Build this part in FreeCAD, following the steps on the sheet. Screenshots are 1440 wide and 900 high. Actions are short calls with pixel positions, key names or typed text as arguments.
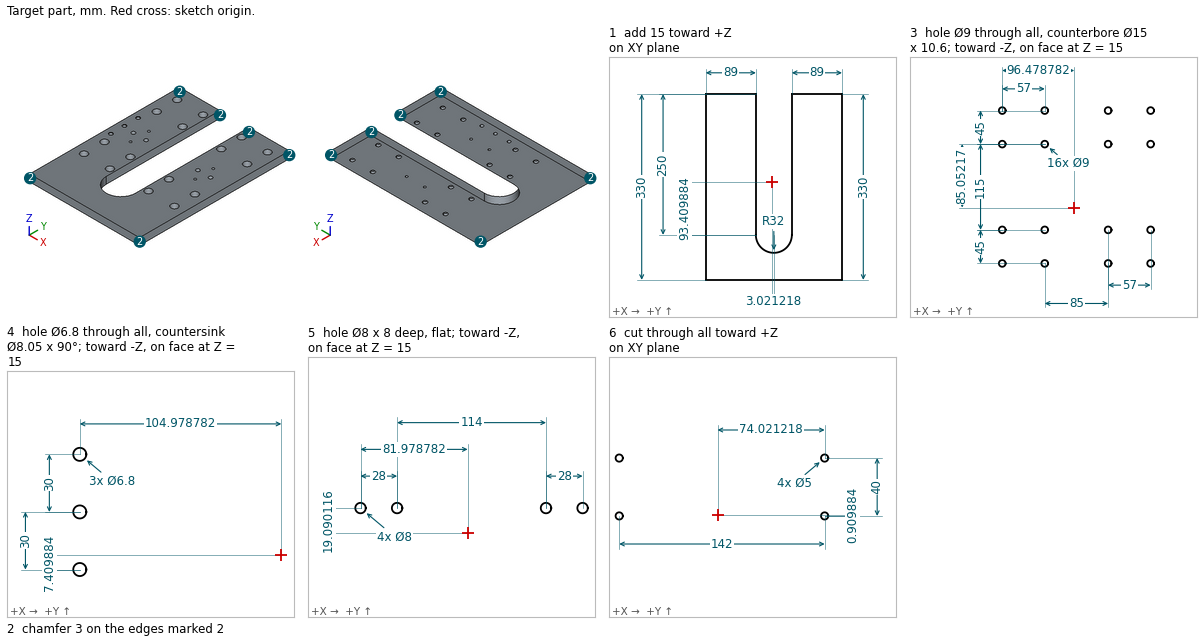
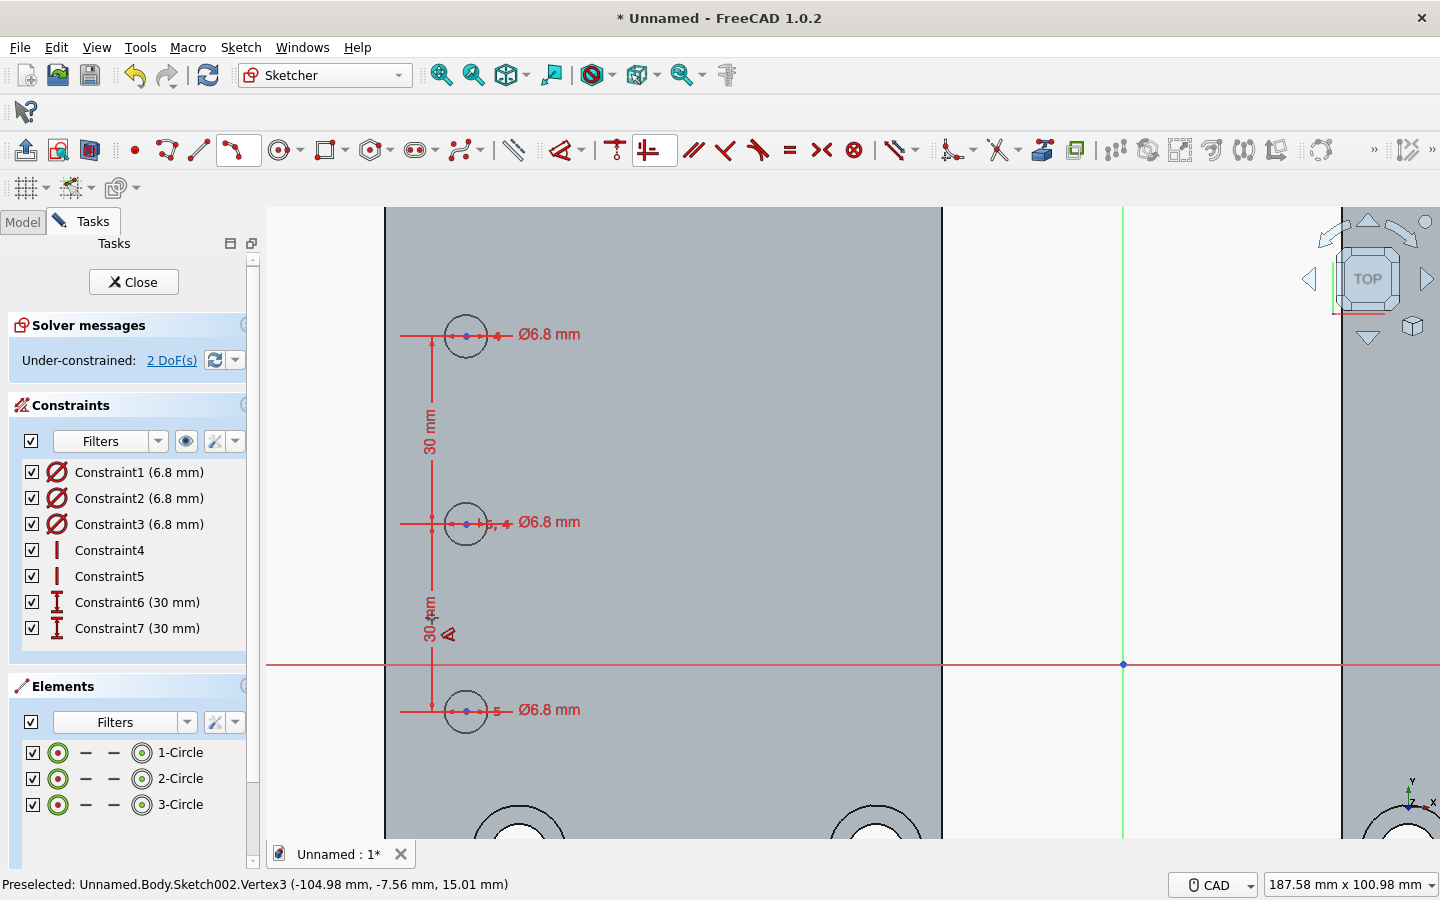
click(466, 712)
click(1157, 688)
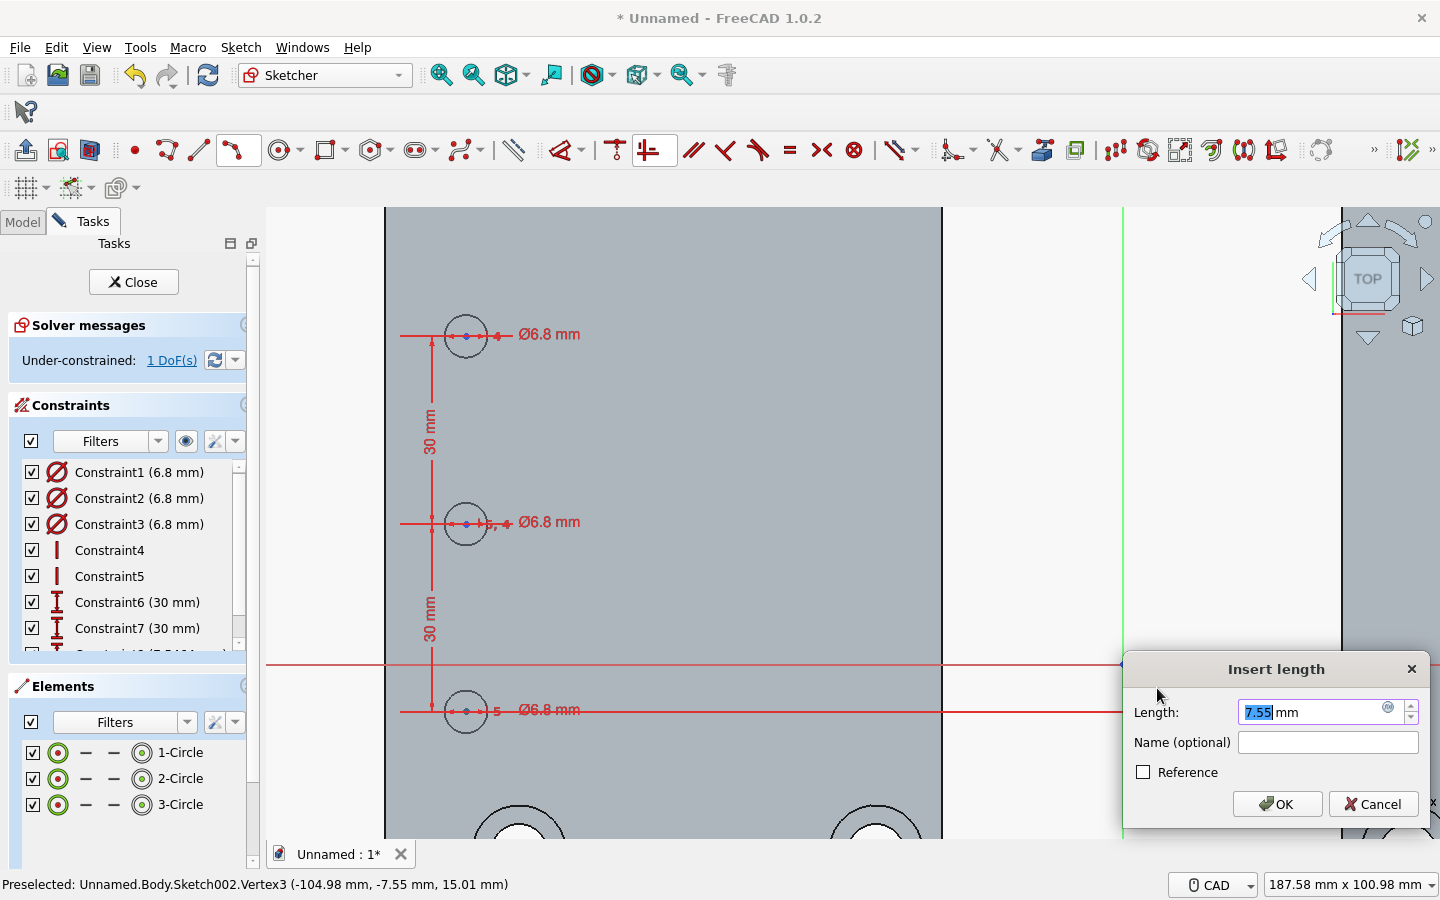
text(7.409884)
key(Return)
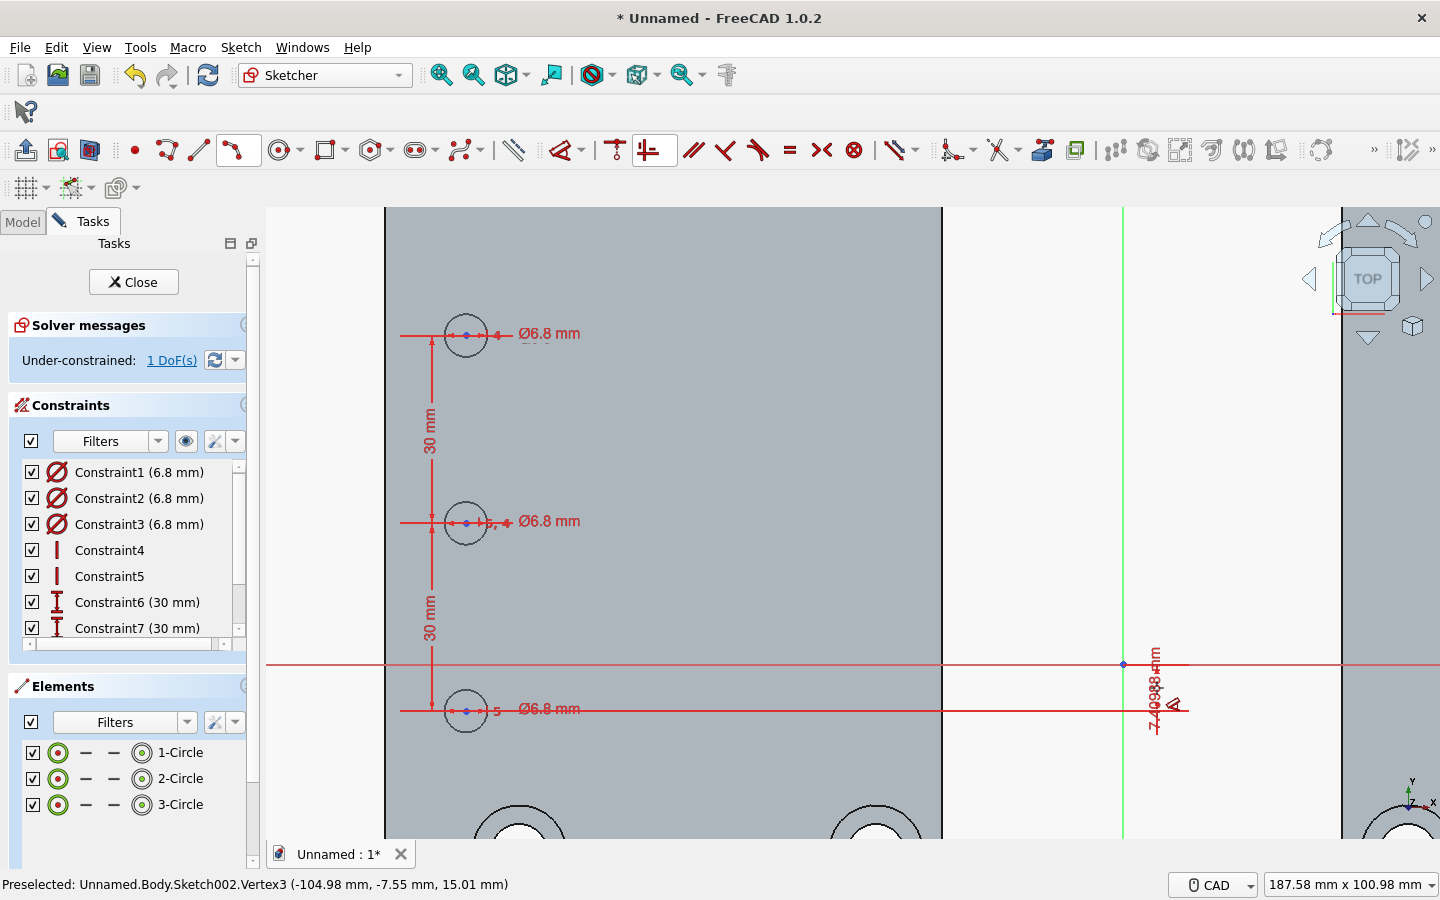
click(466, 336)
click(795, 302)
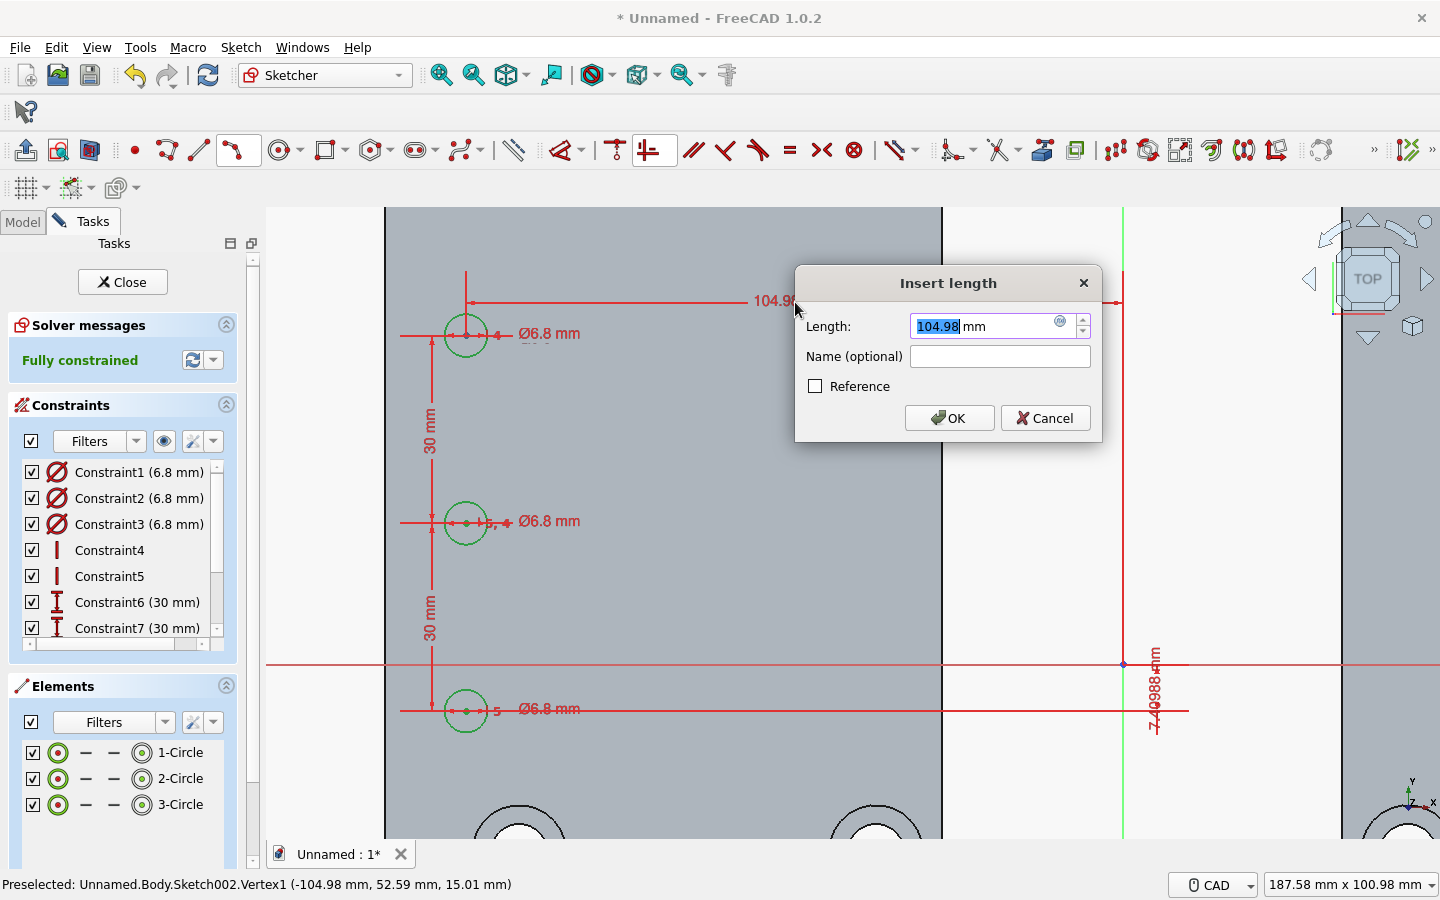
text(104.978782)
key(Return)
key(Escape)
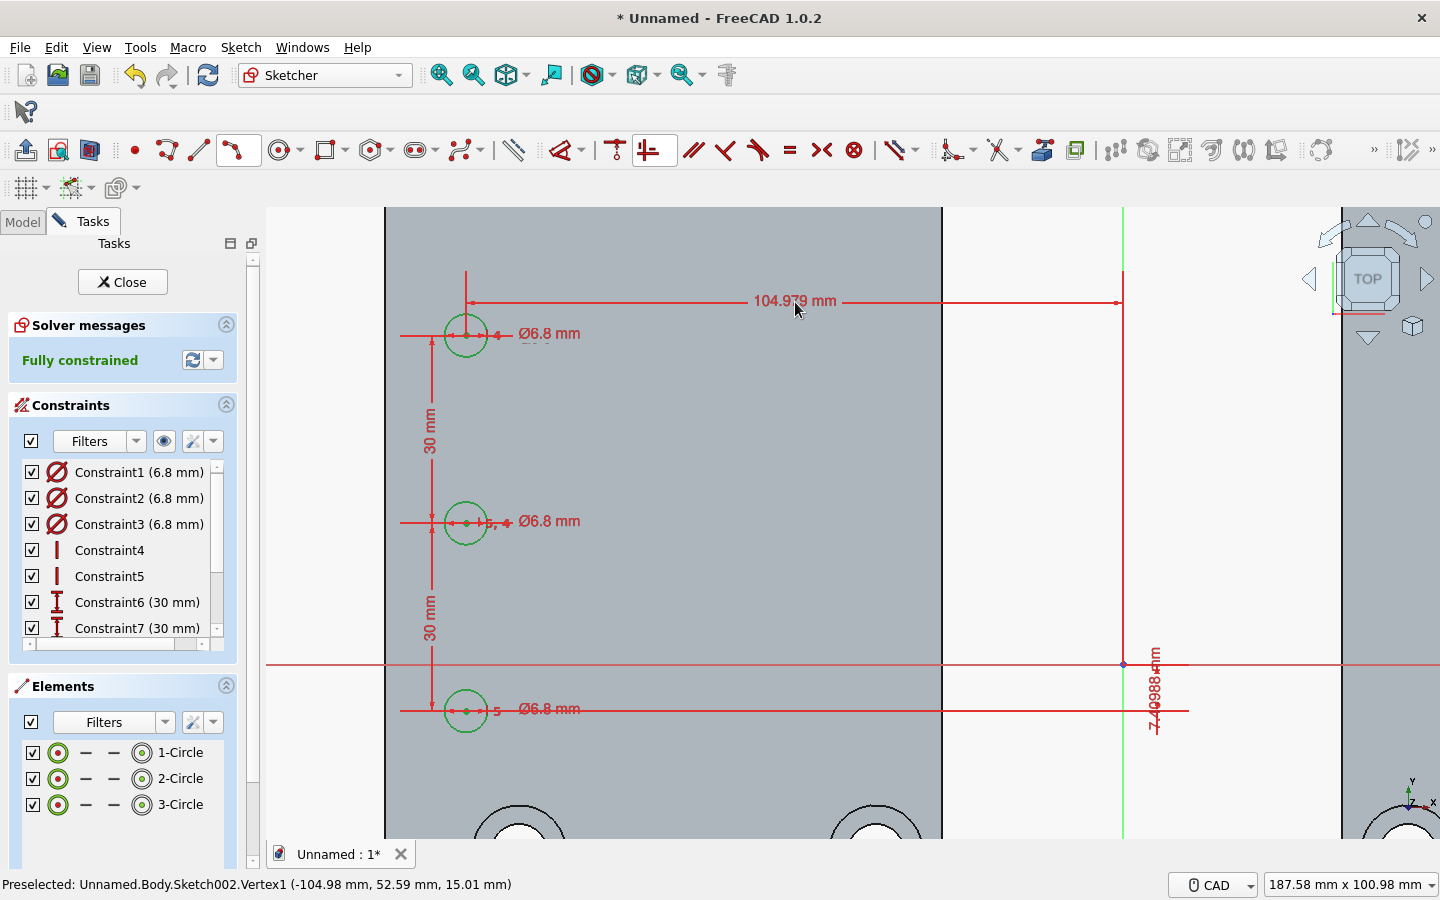
click(123, 282)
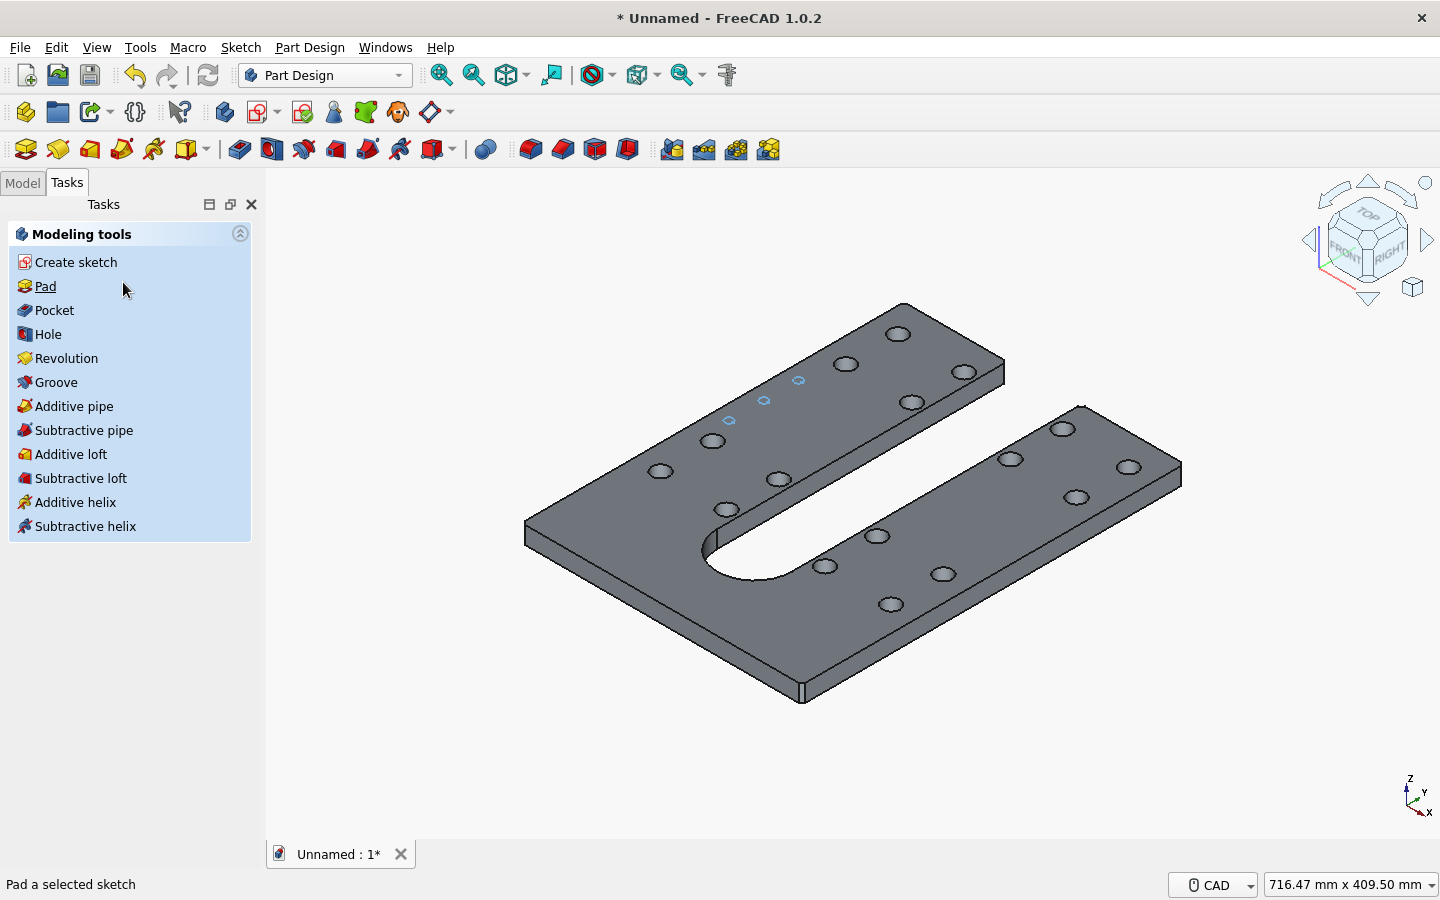
click(272, 150)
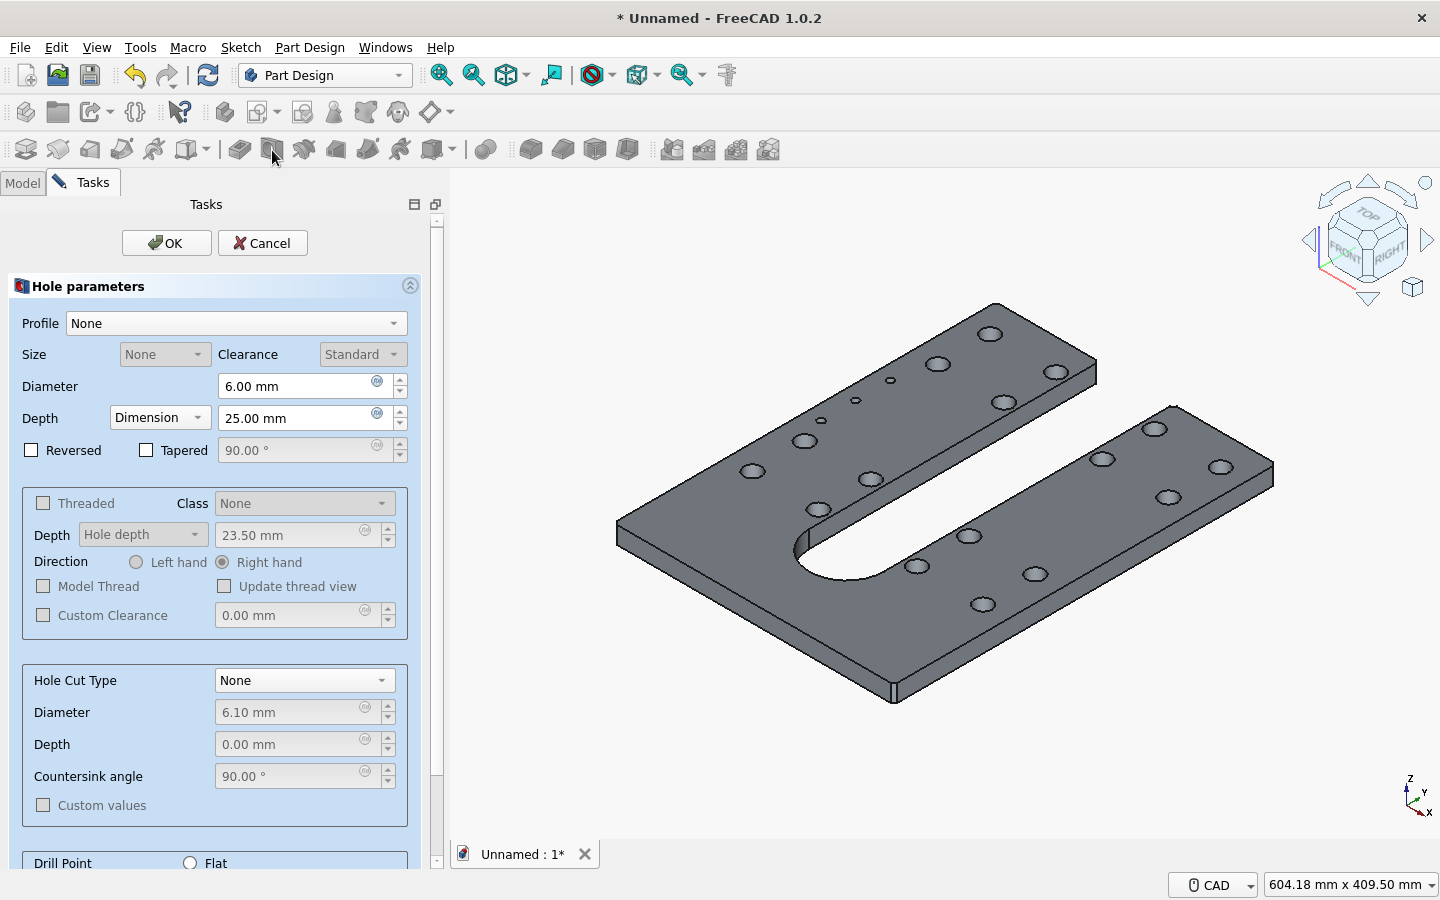
triple_click(305, 386)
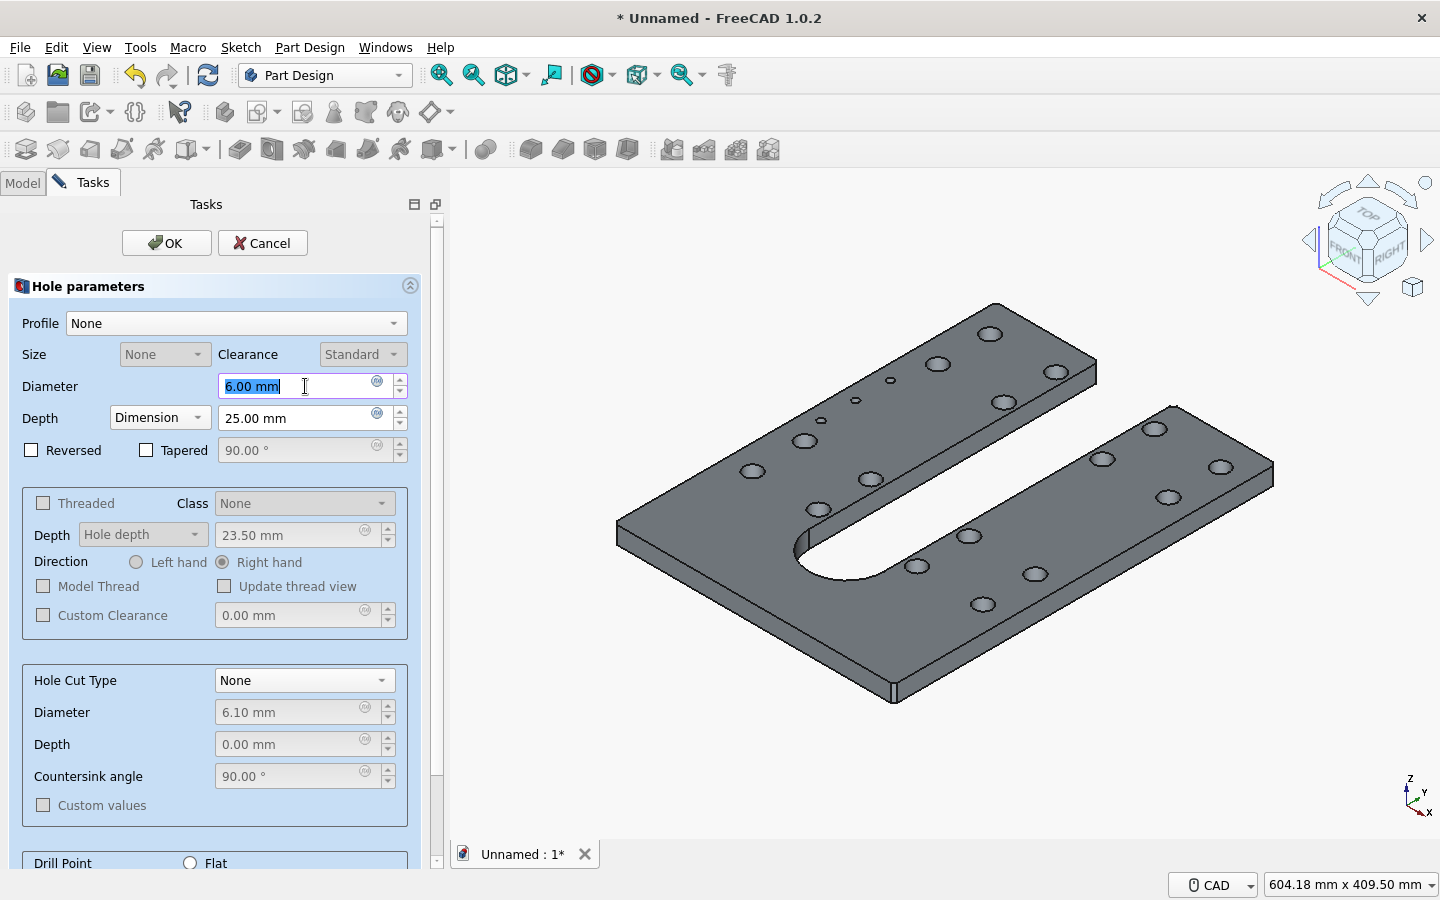
text(6.8)
key(Tab)